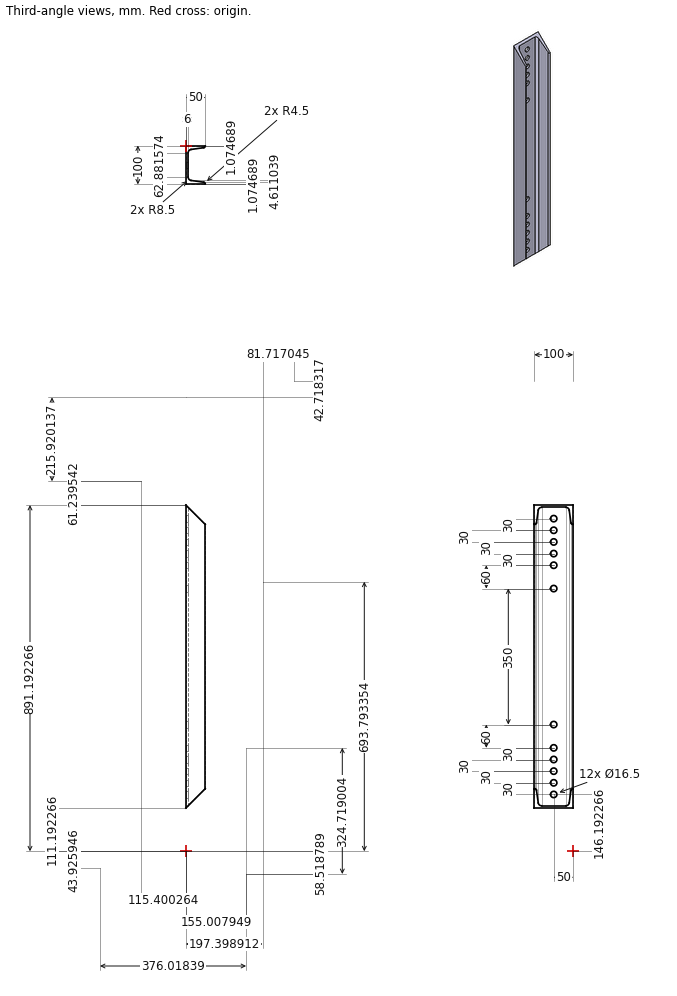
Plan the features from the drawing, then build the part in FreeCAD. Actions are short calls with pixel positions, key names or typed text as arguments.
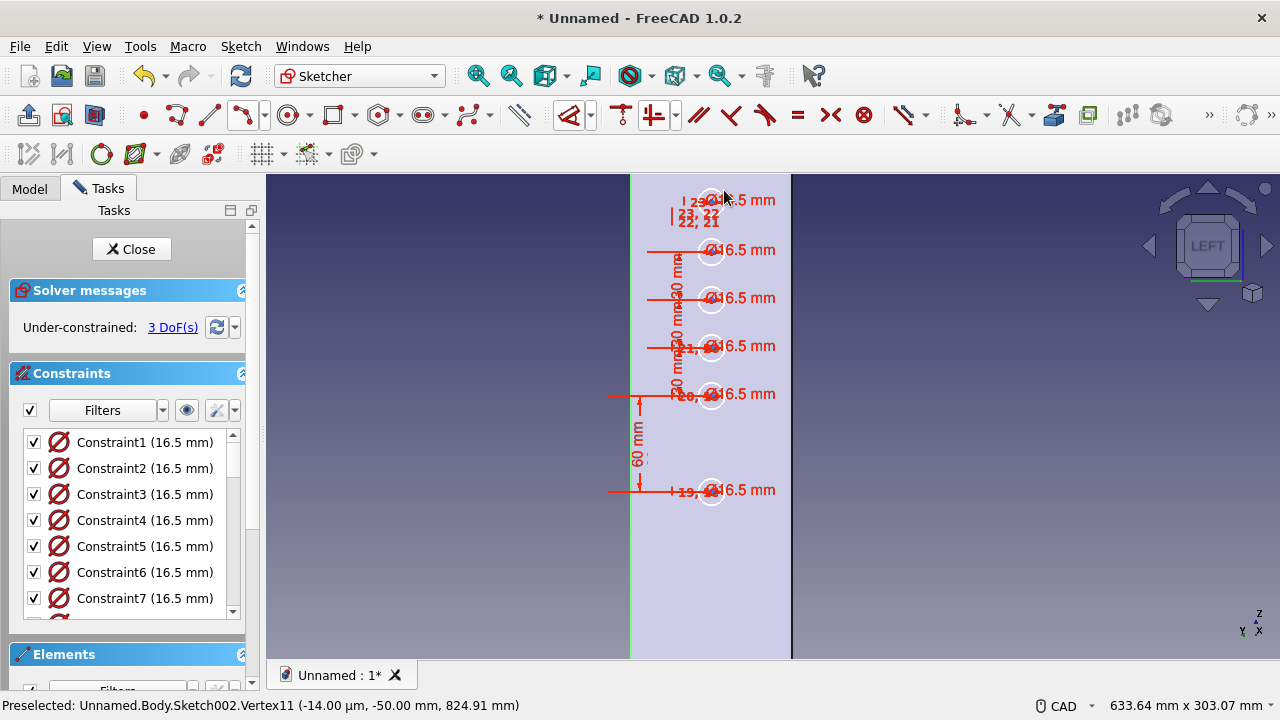
click(712, 252)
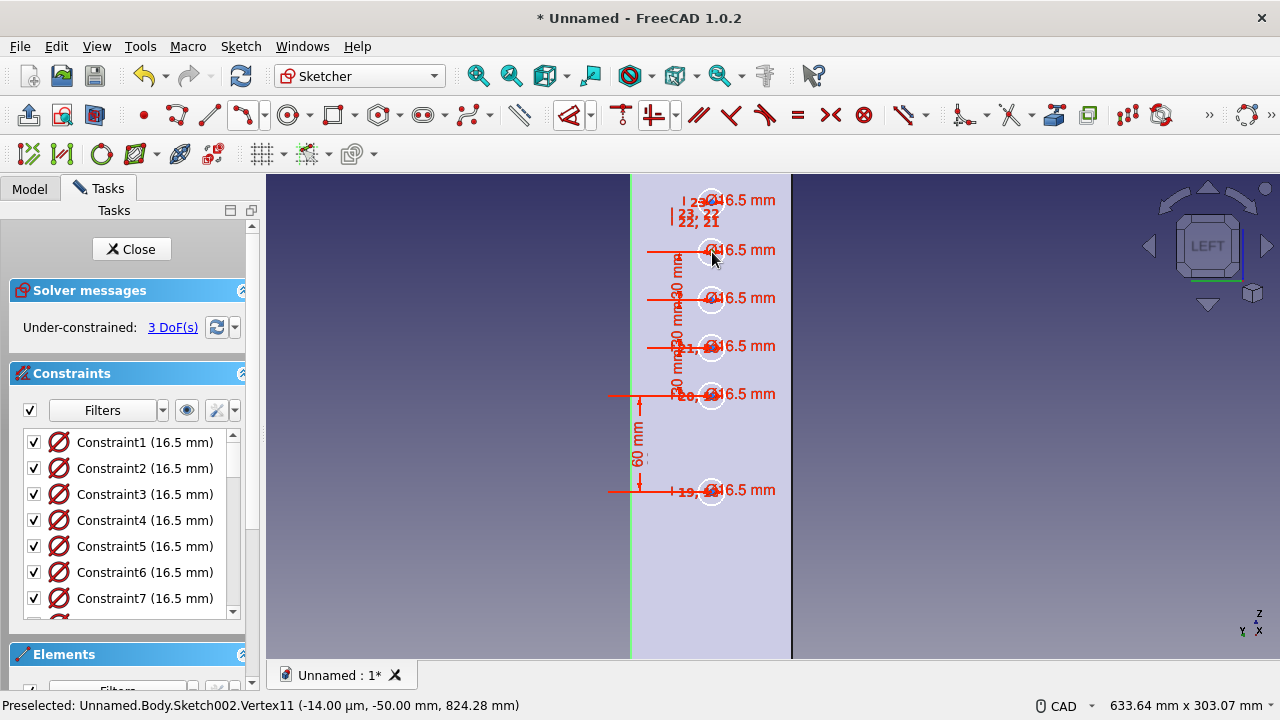
click(712, 202)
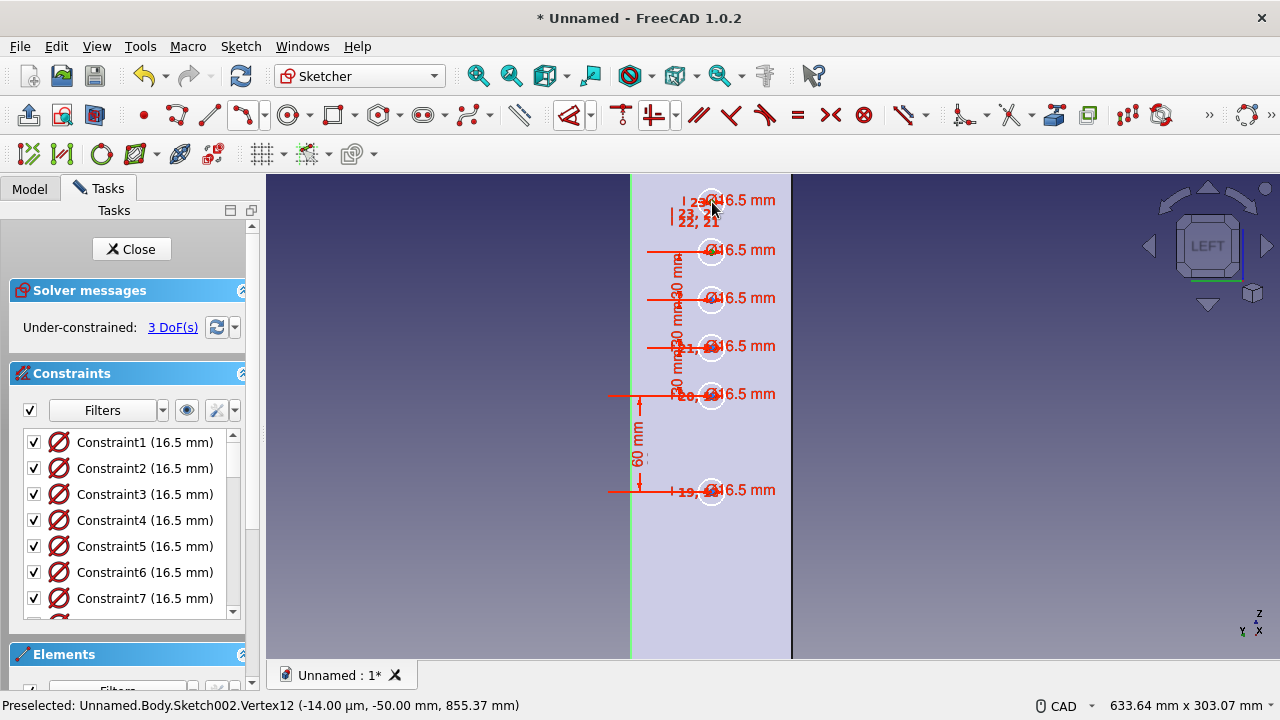
click(590, 116)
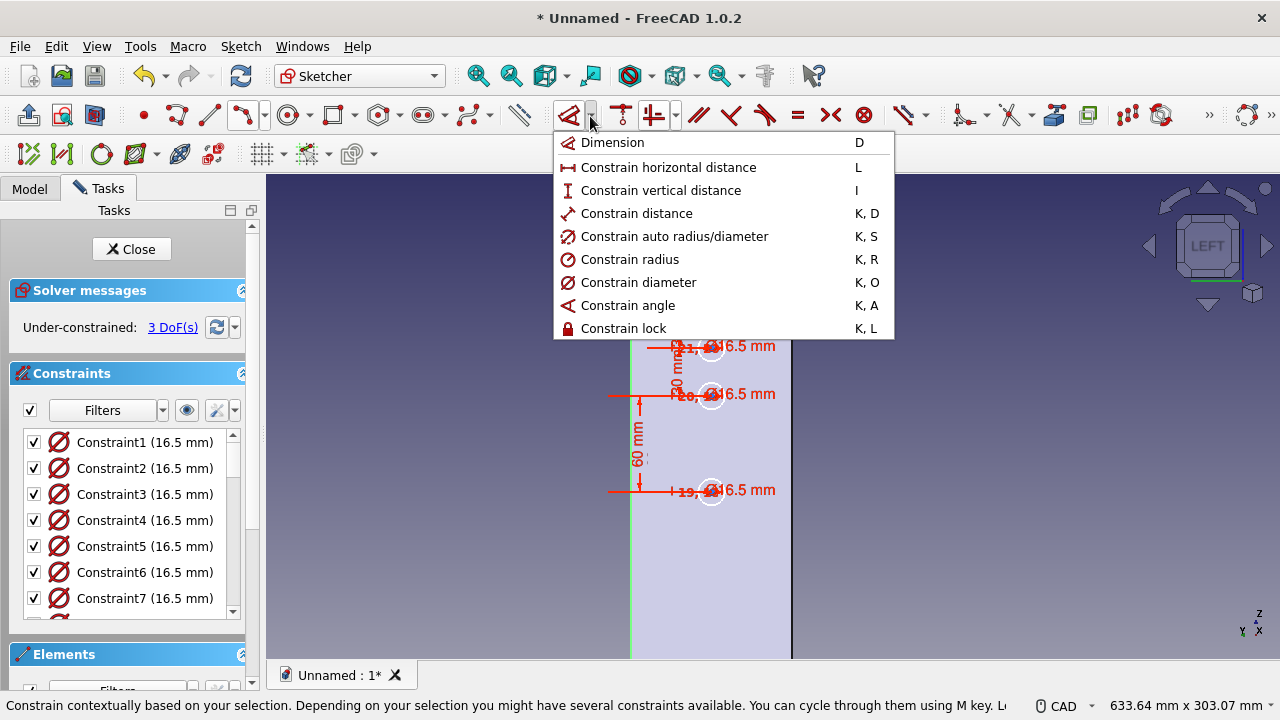
click(724, 190)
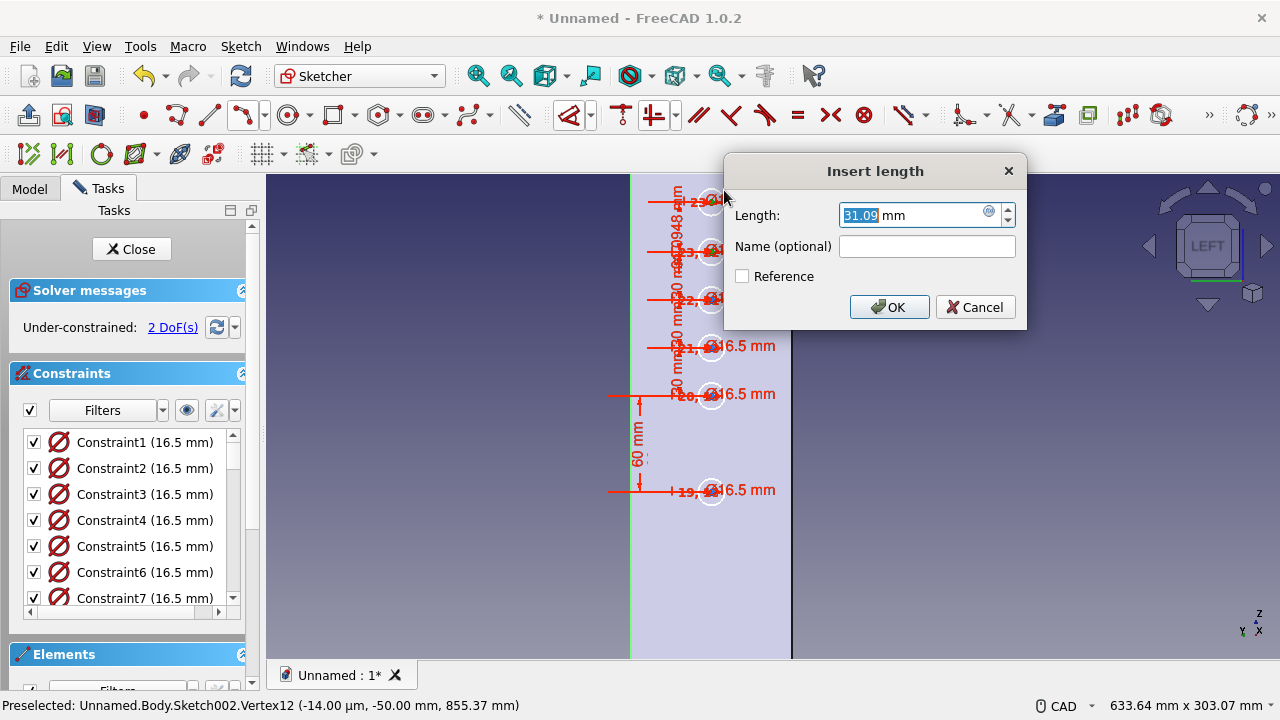
text(30)
key(Return)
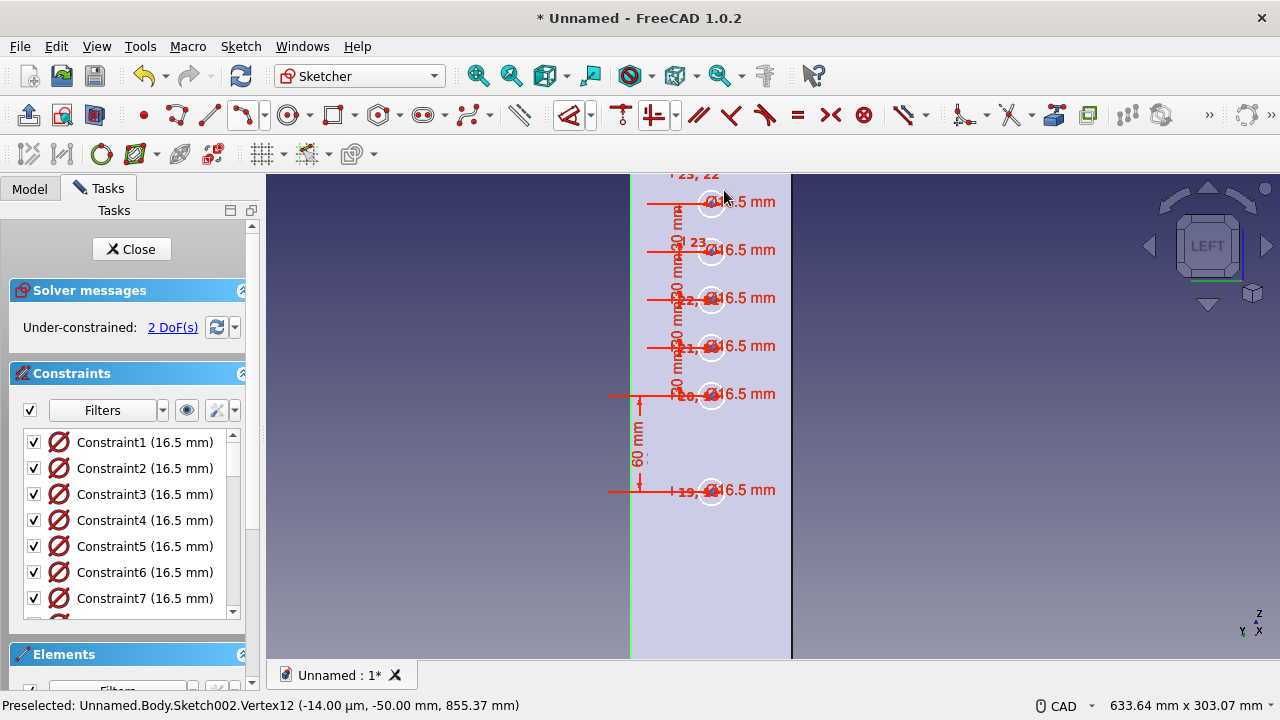
scroll(711, 299, down, 8)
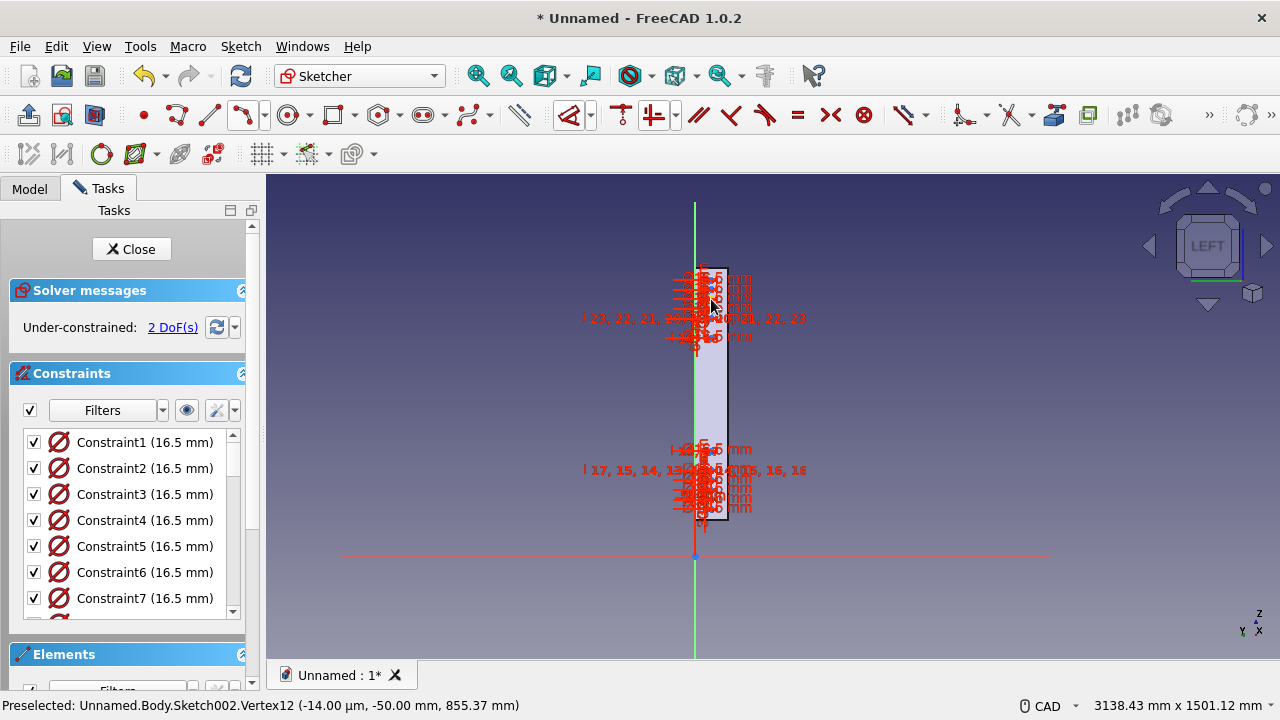
click(711, 451)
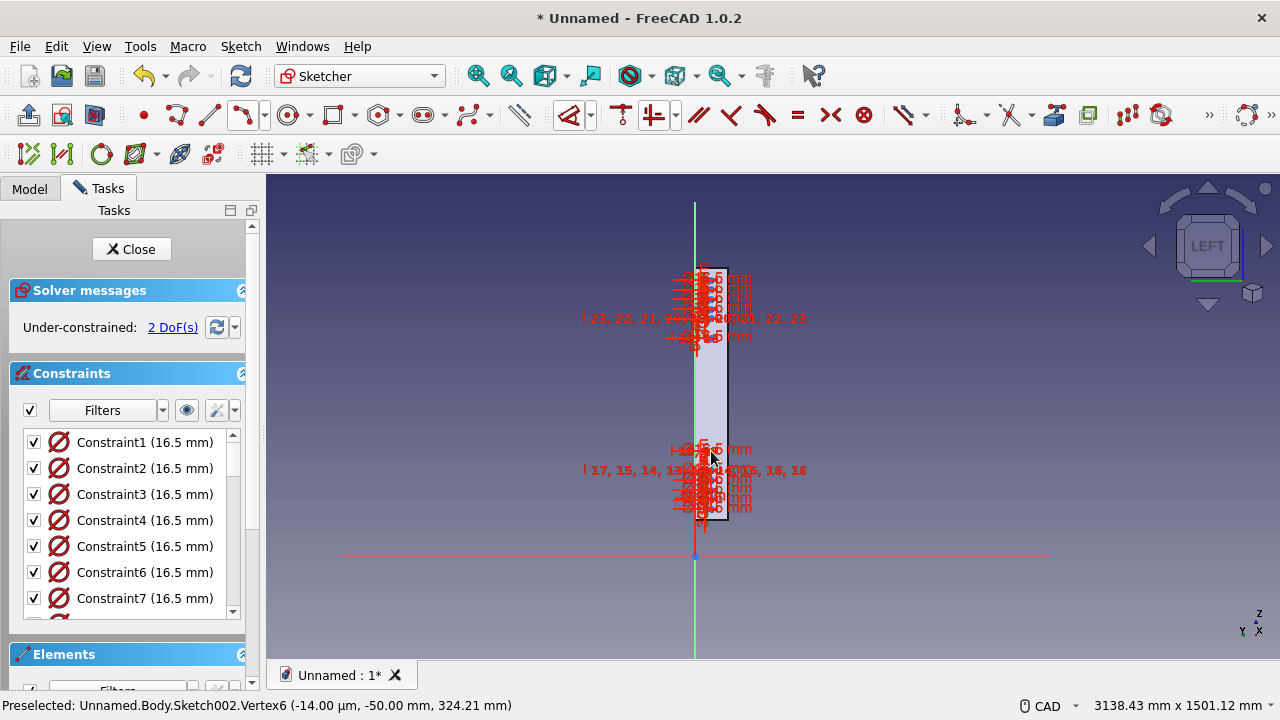
click(711, 338)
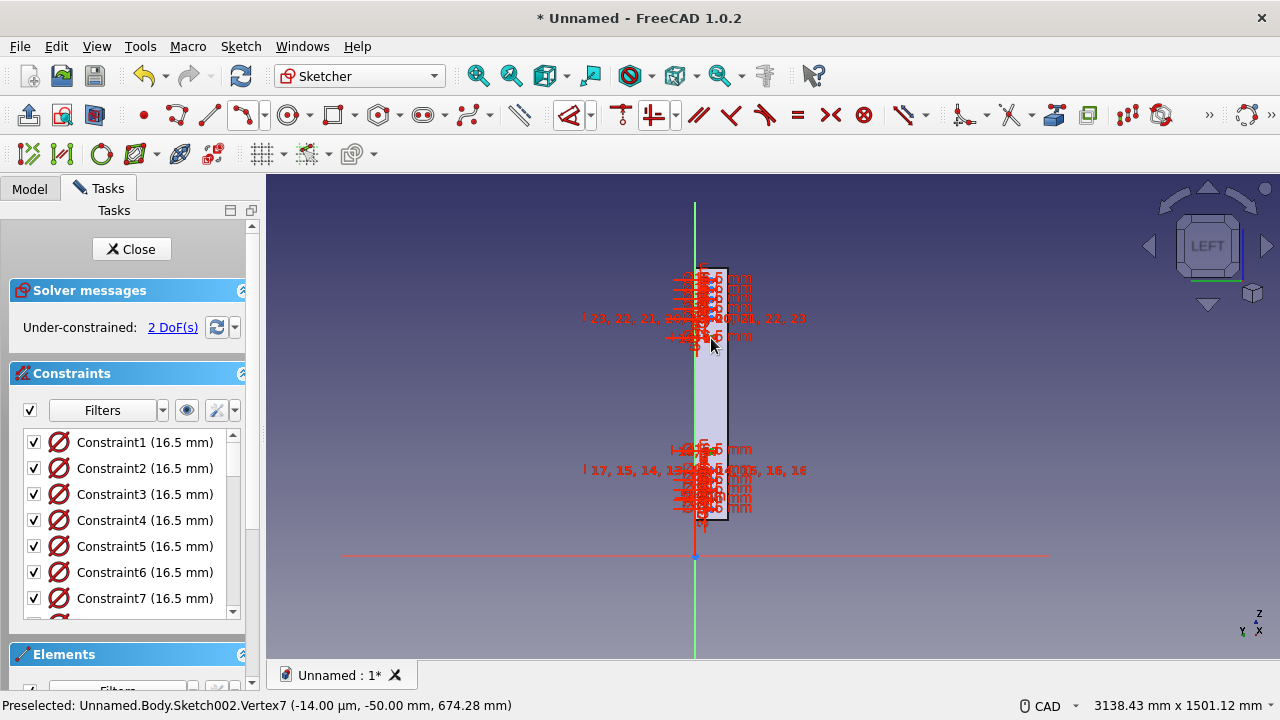
key(i)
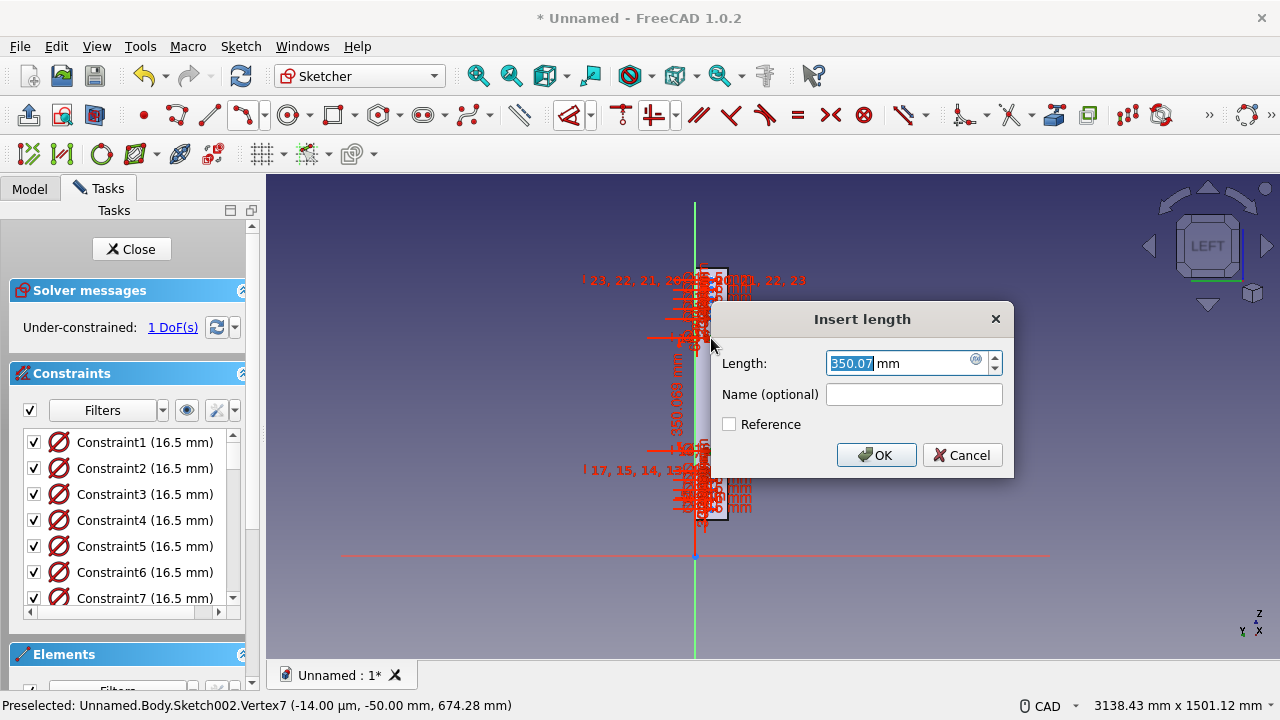
text(350)
key(Return)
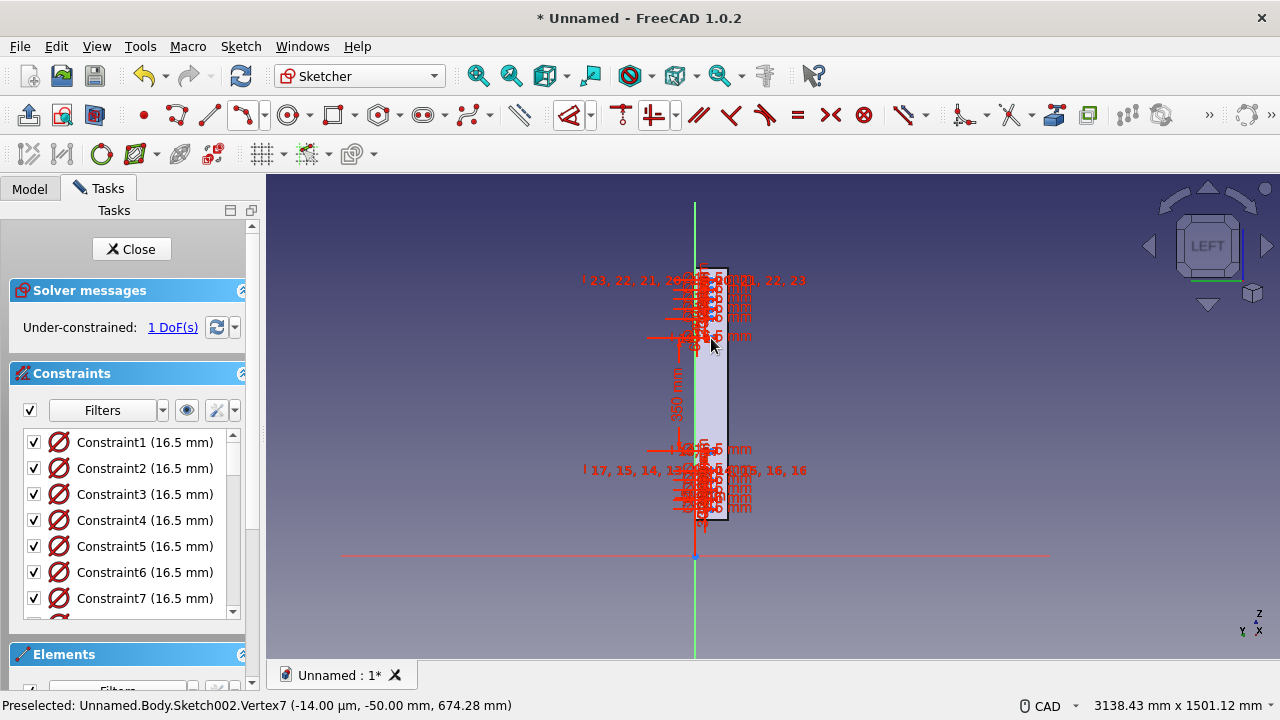
scroll(711, 509, up, 2)